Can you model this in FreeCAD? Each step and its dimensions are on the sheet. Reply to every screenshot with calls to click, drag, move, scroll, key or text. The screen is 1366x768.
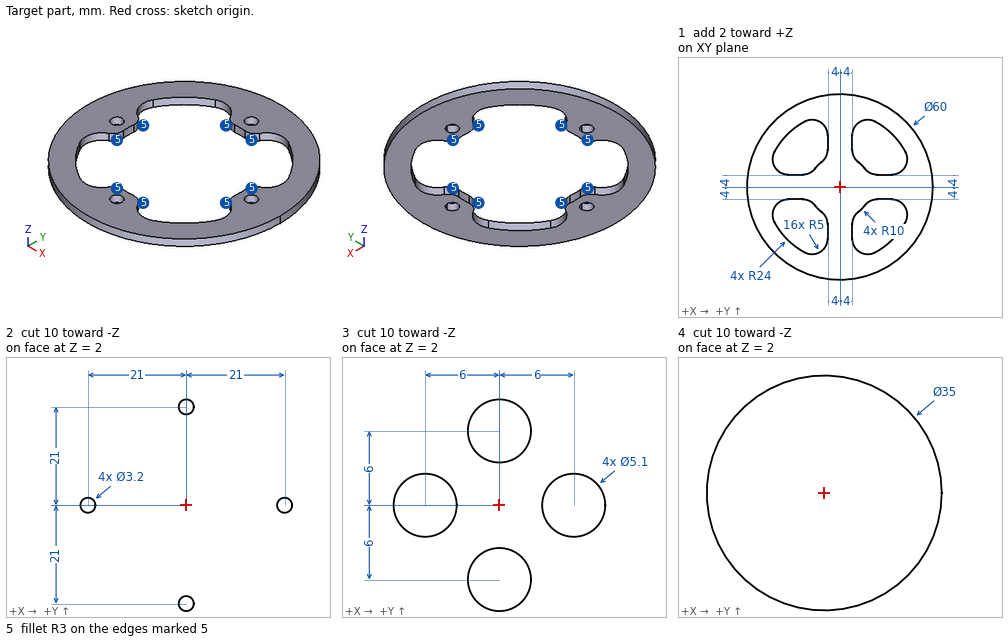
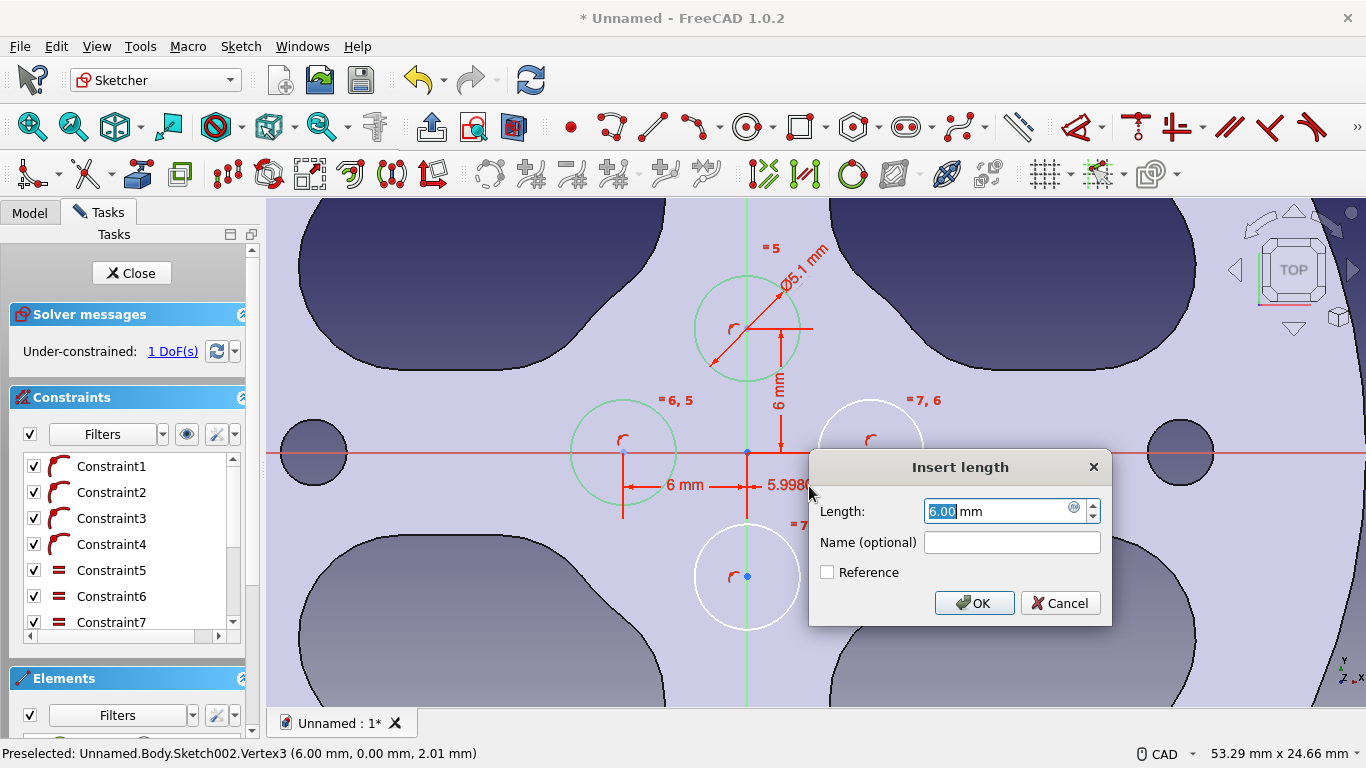
text(6)
key(Return)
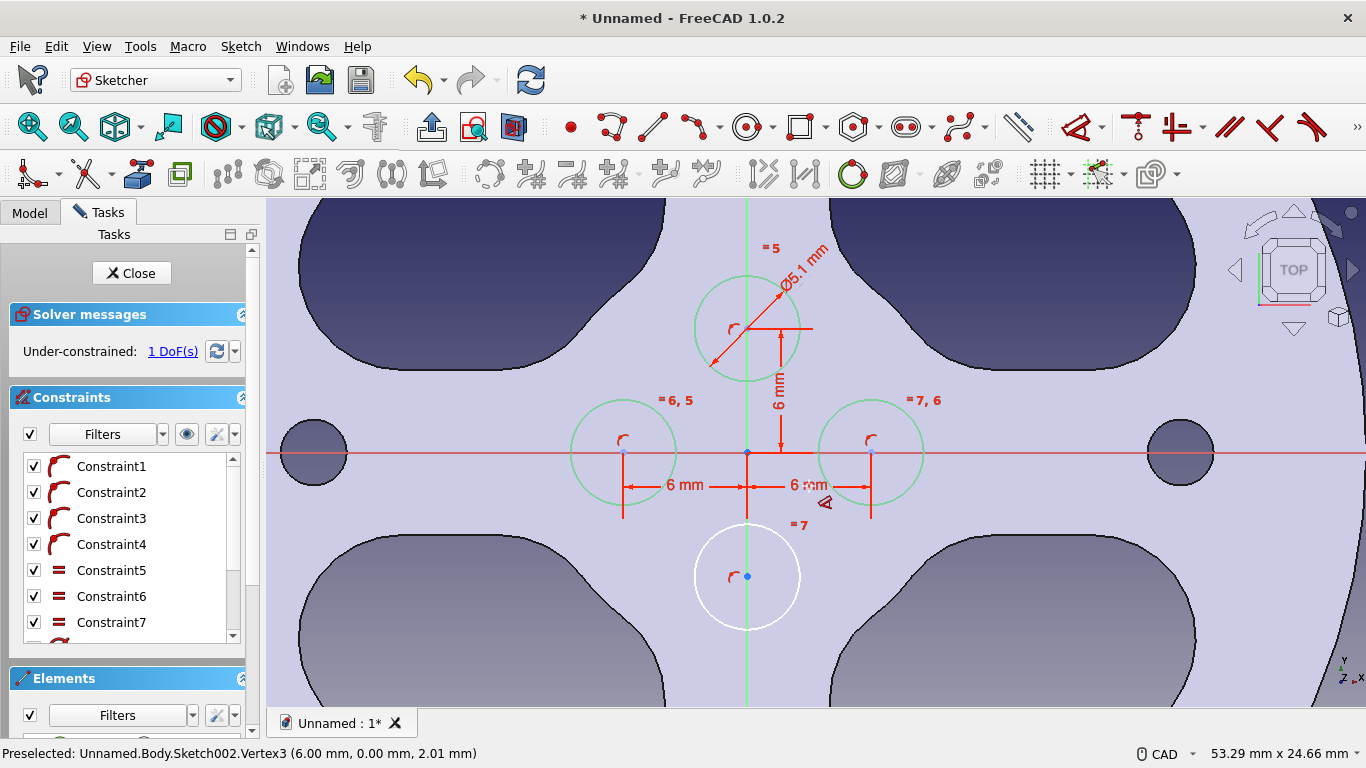
click(747, 577)
click(781, 515)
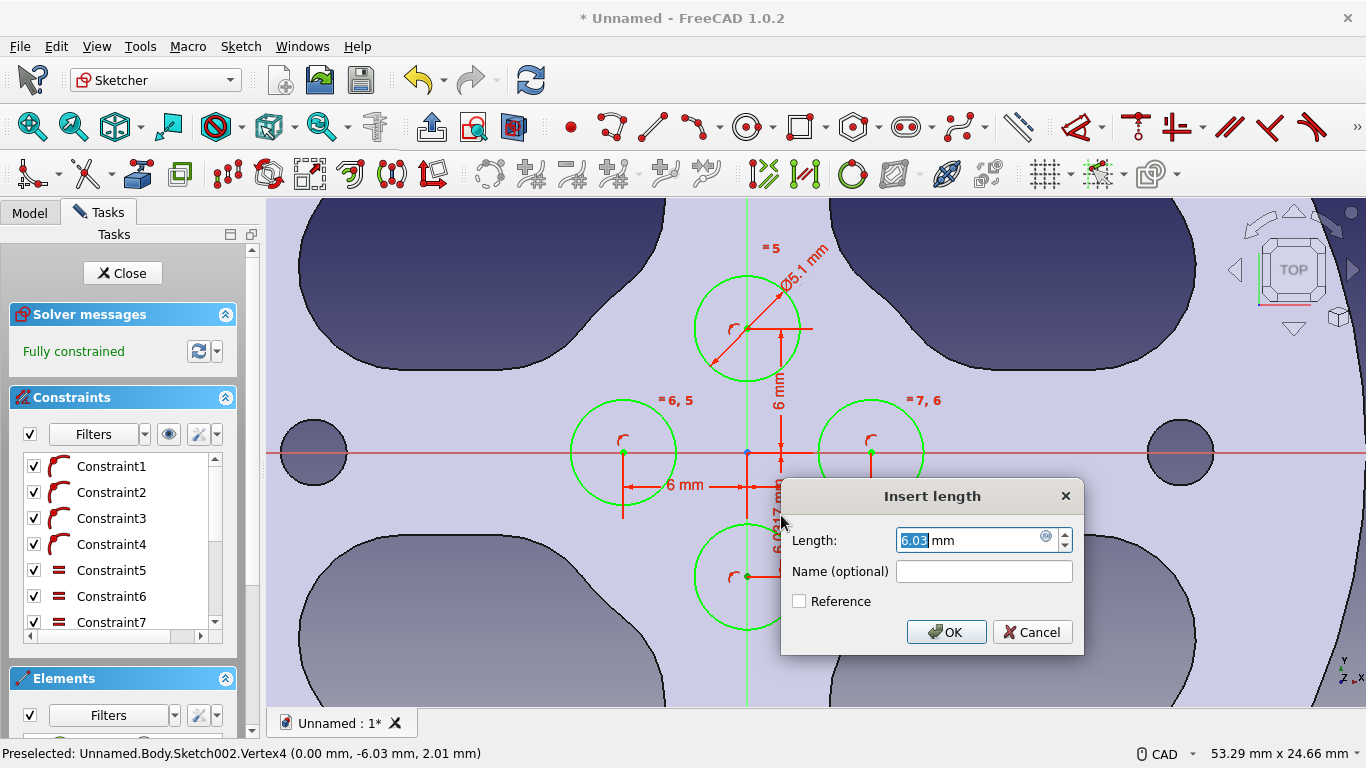
text(6)
key(Return)
key(Escape)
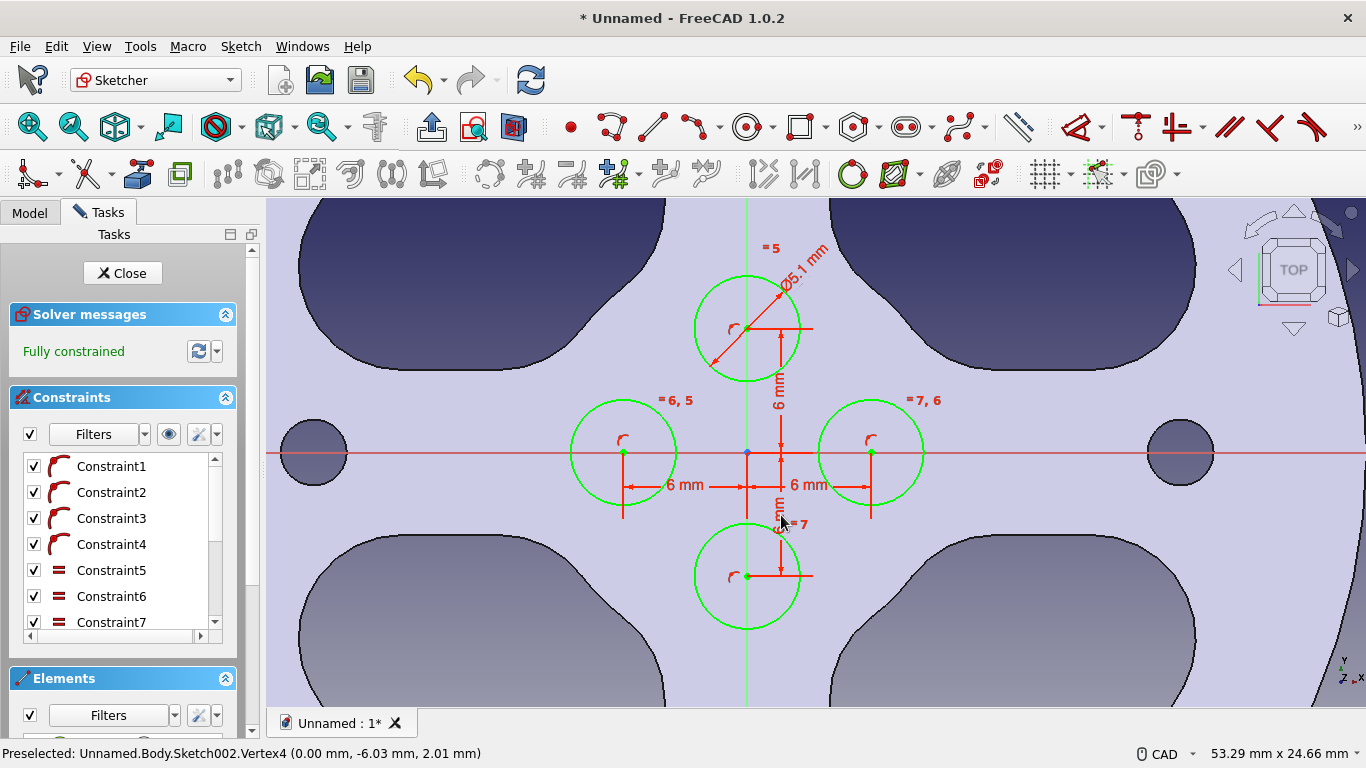
click(123, 273)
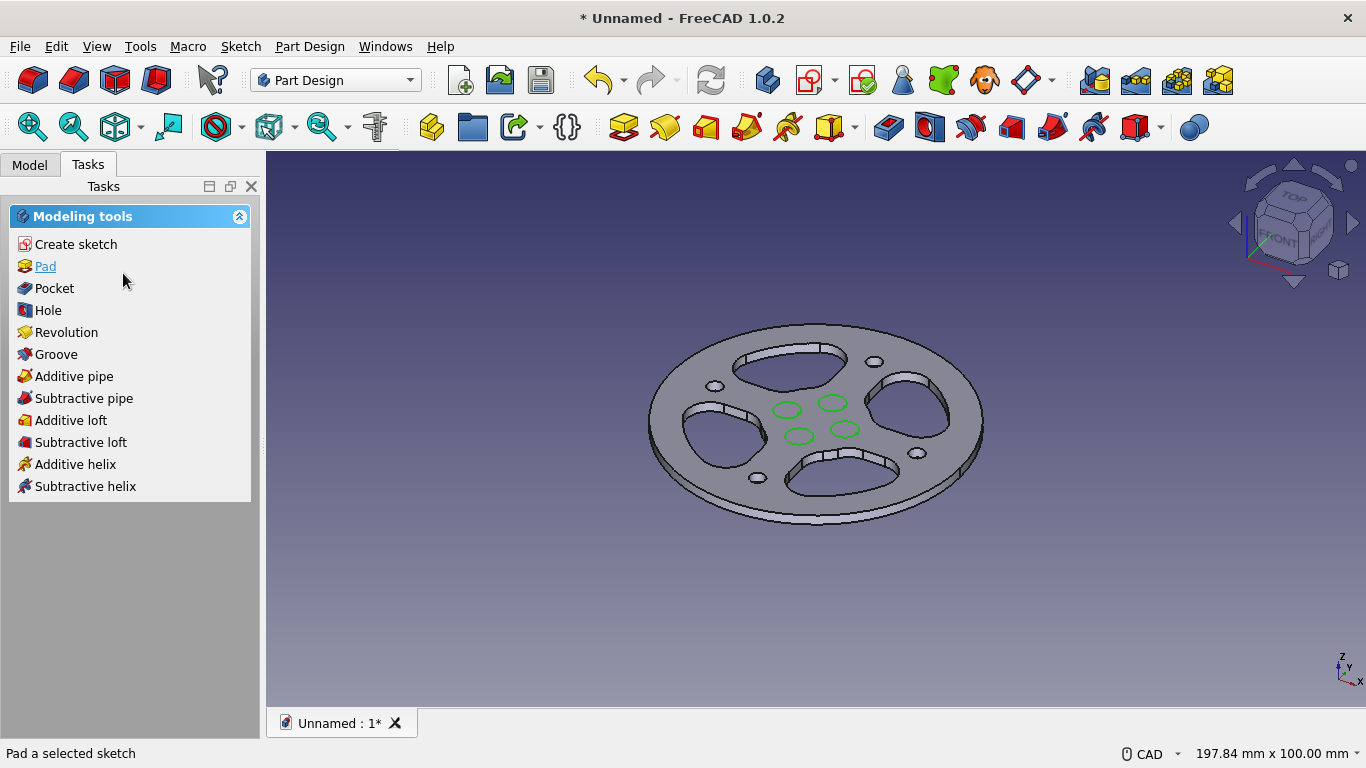
click(889, 128)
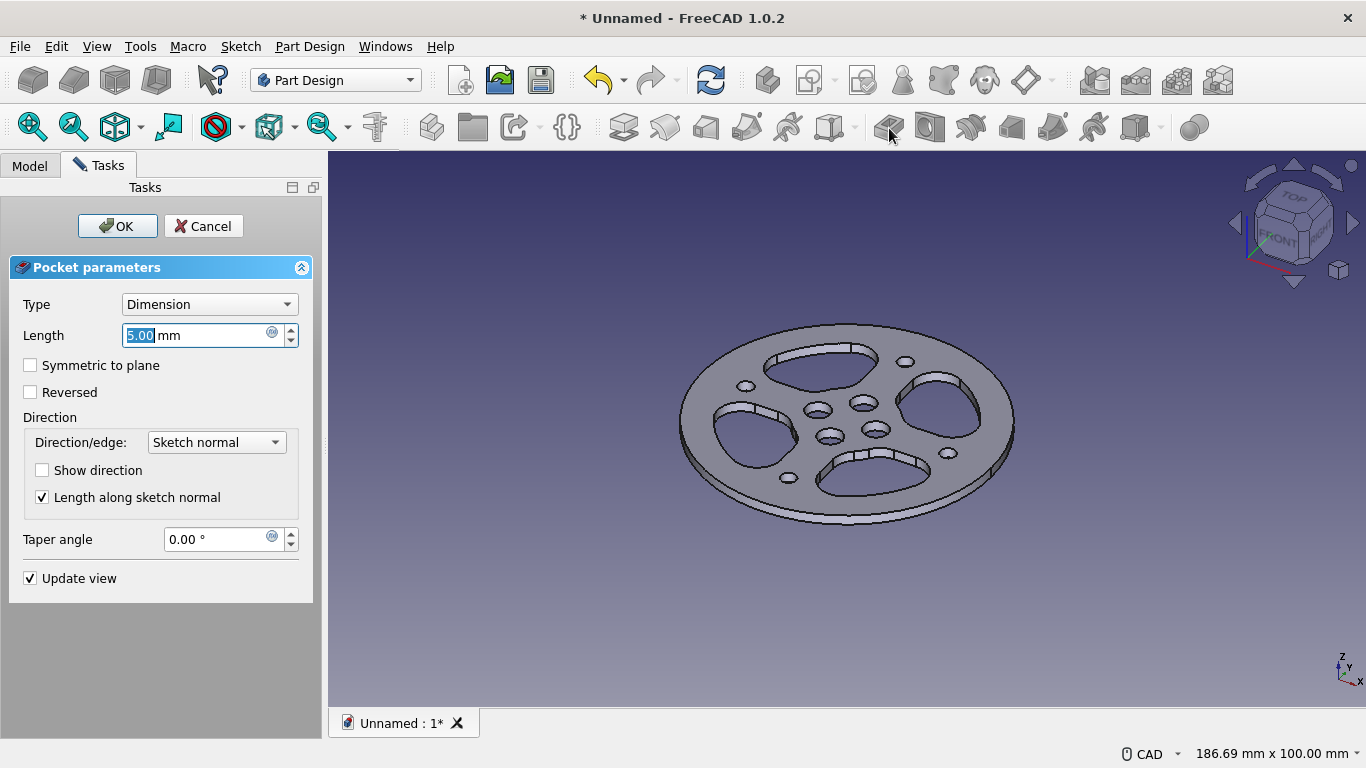
text(10)
key(Tab)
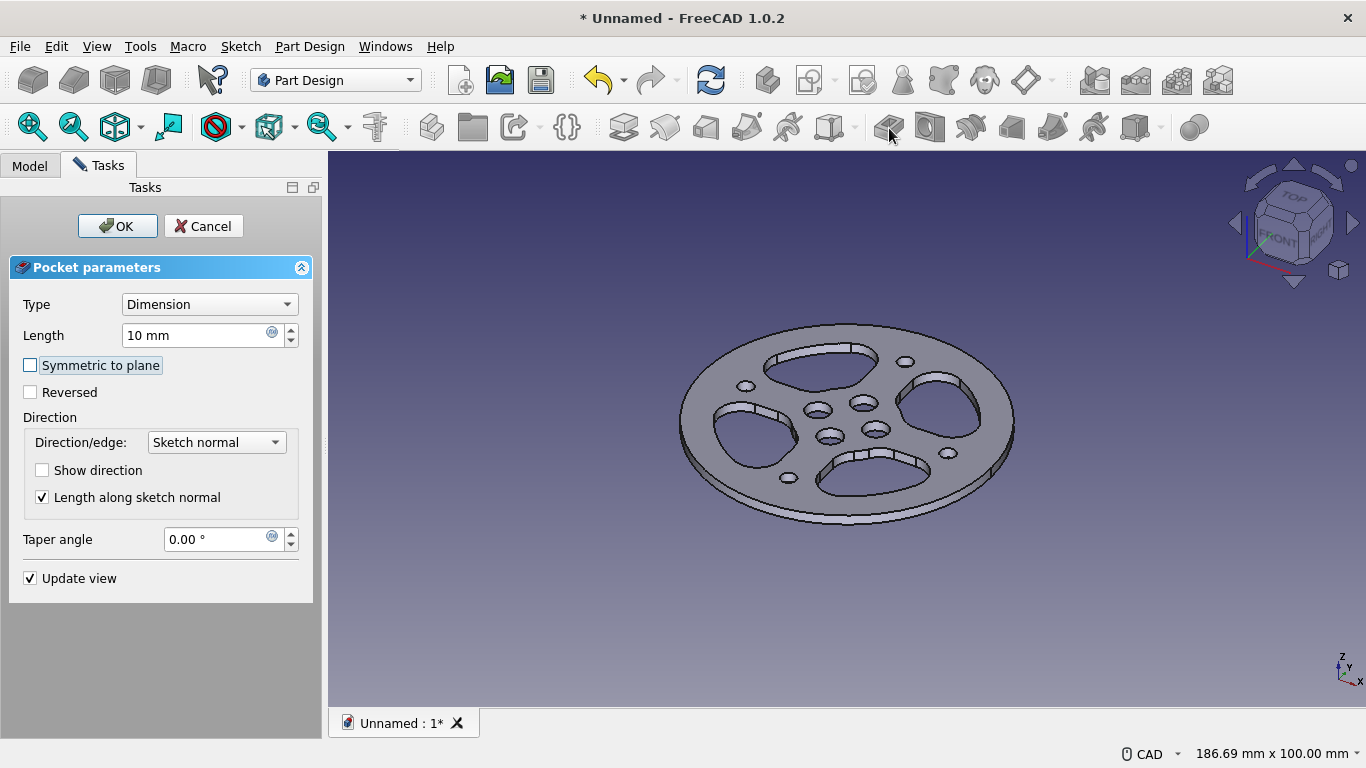
click(118, 226)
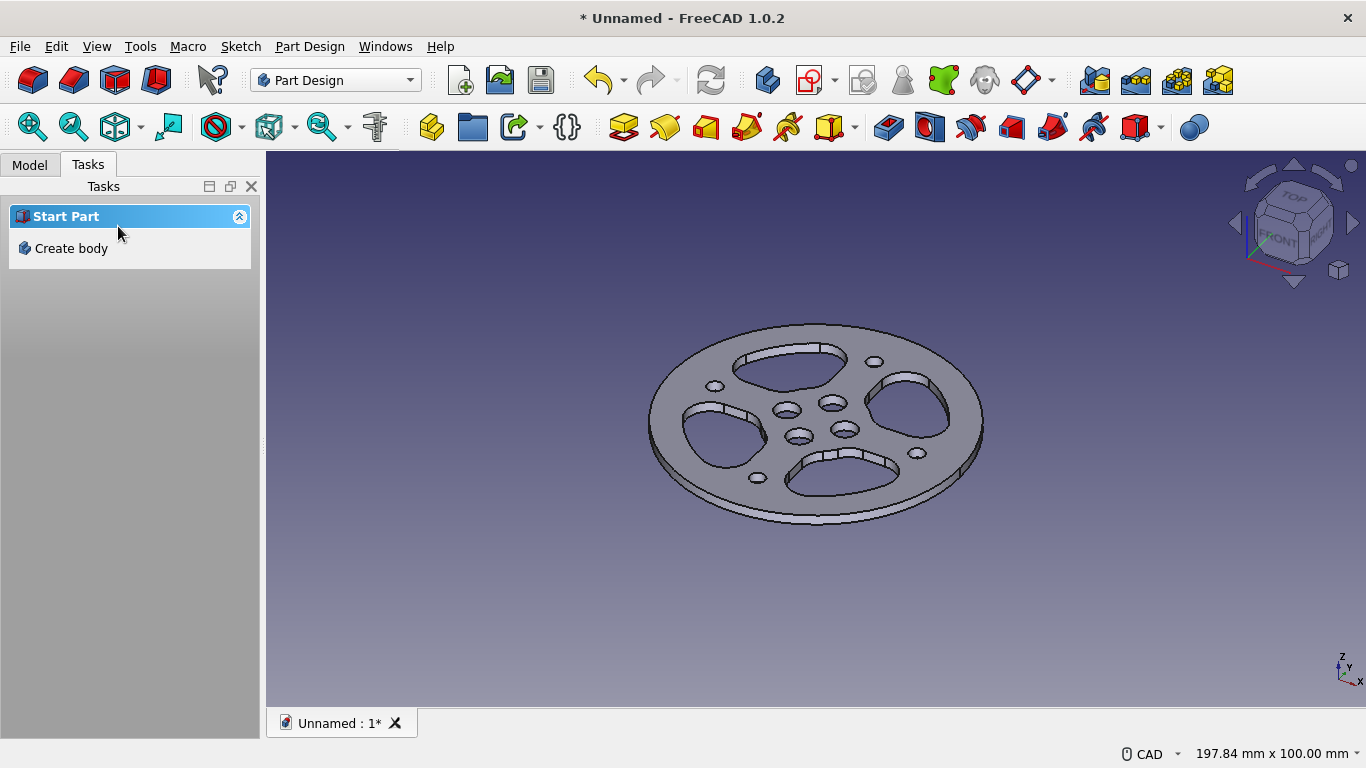
click(816, 419)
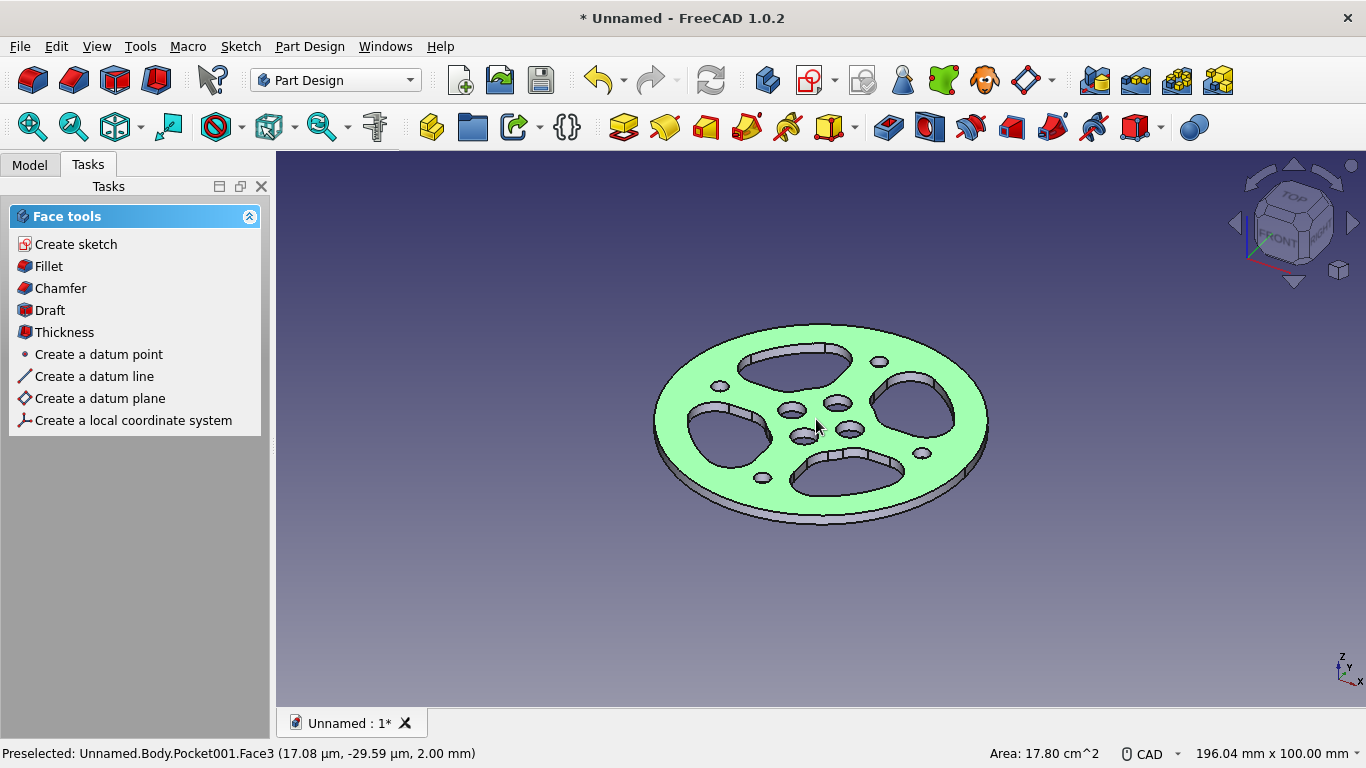
click(808, 80)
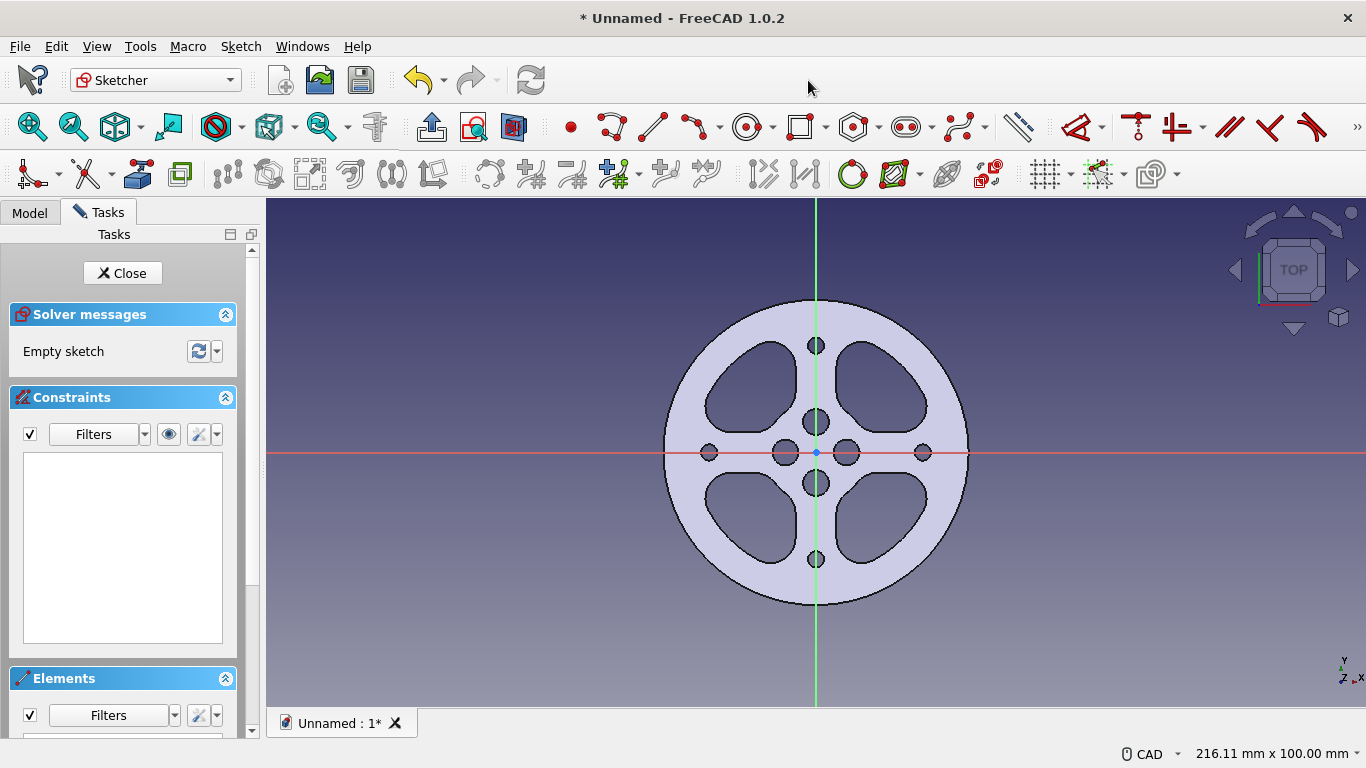
scroll(899, 452, up, 3)